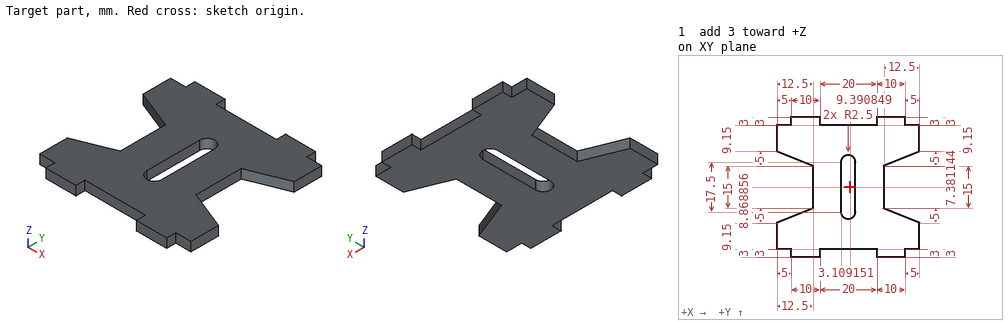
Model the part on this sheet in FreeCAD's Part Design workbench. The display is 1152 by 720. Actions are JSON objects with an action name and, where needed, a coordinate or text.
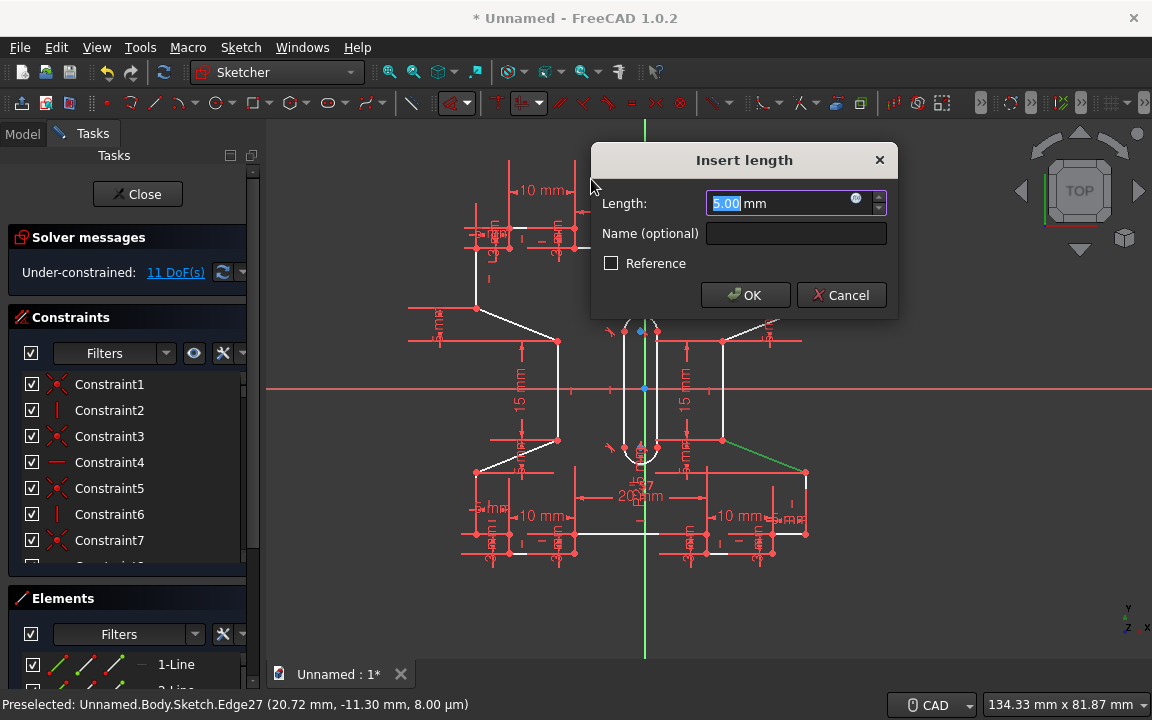
{"action": "type", "text": "5"}
{"action": "key", "text": "Return"}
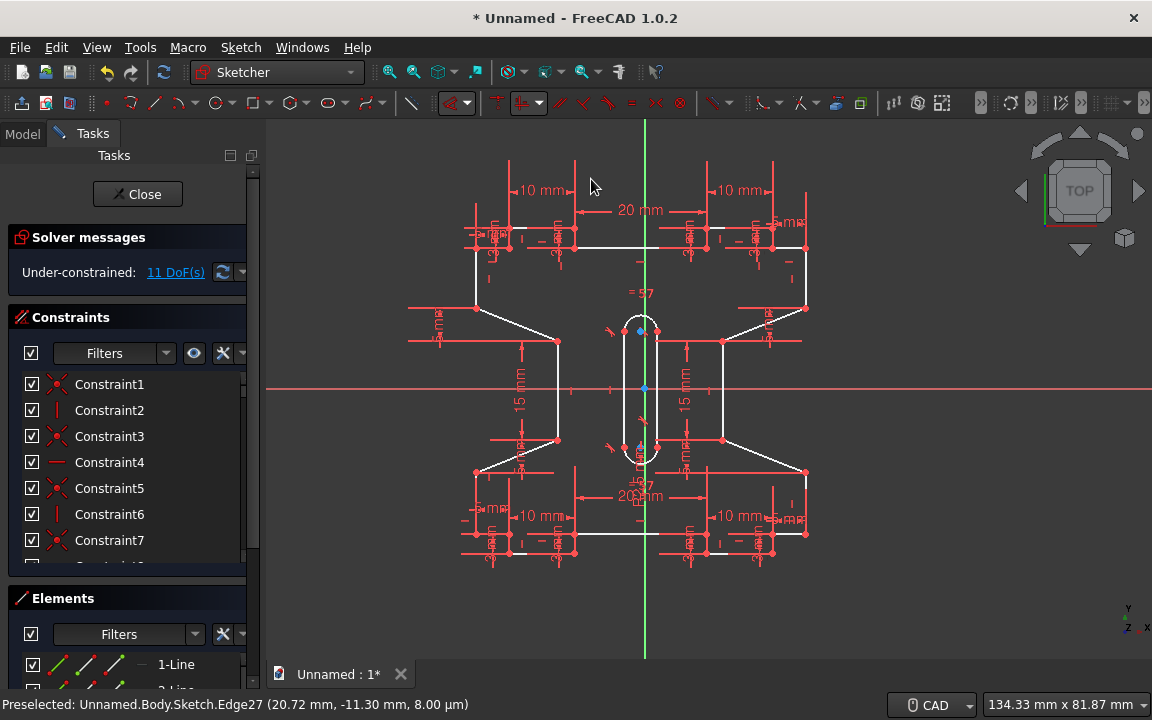
{"action": "left_click", "coordinate": [806, 290]}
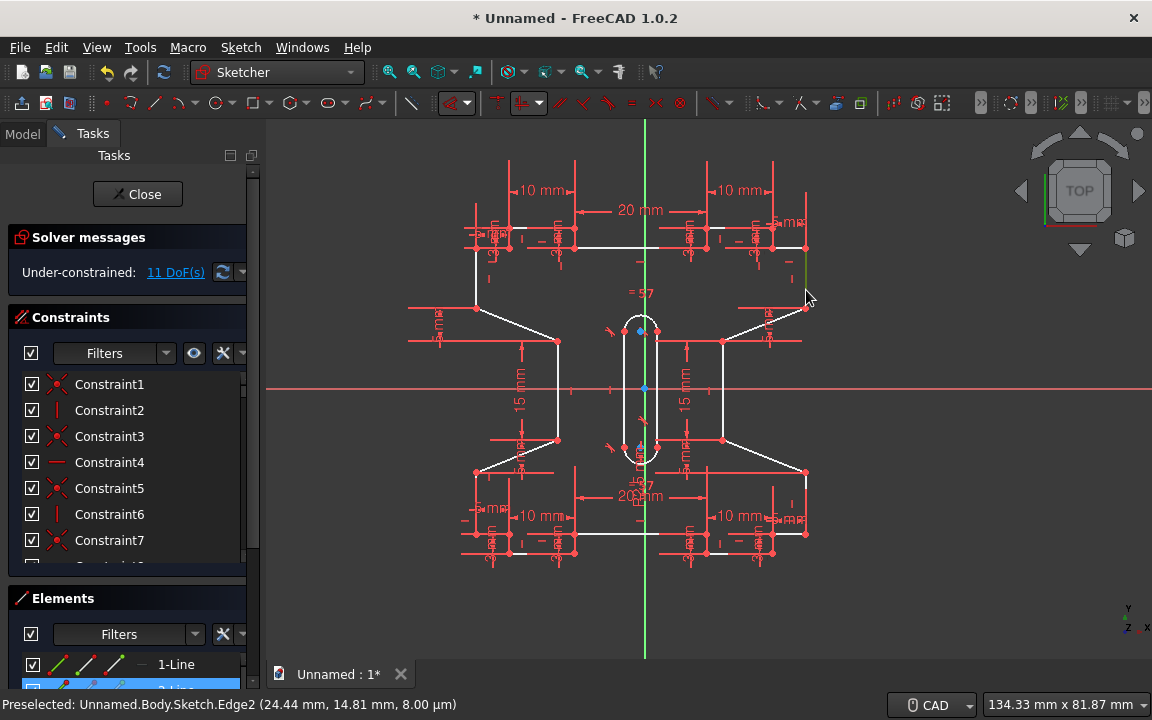
{"action": "left_click", "coordinate": [470, 104]}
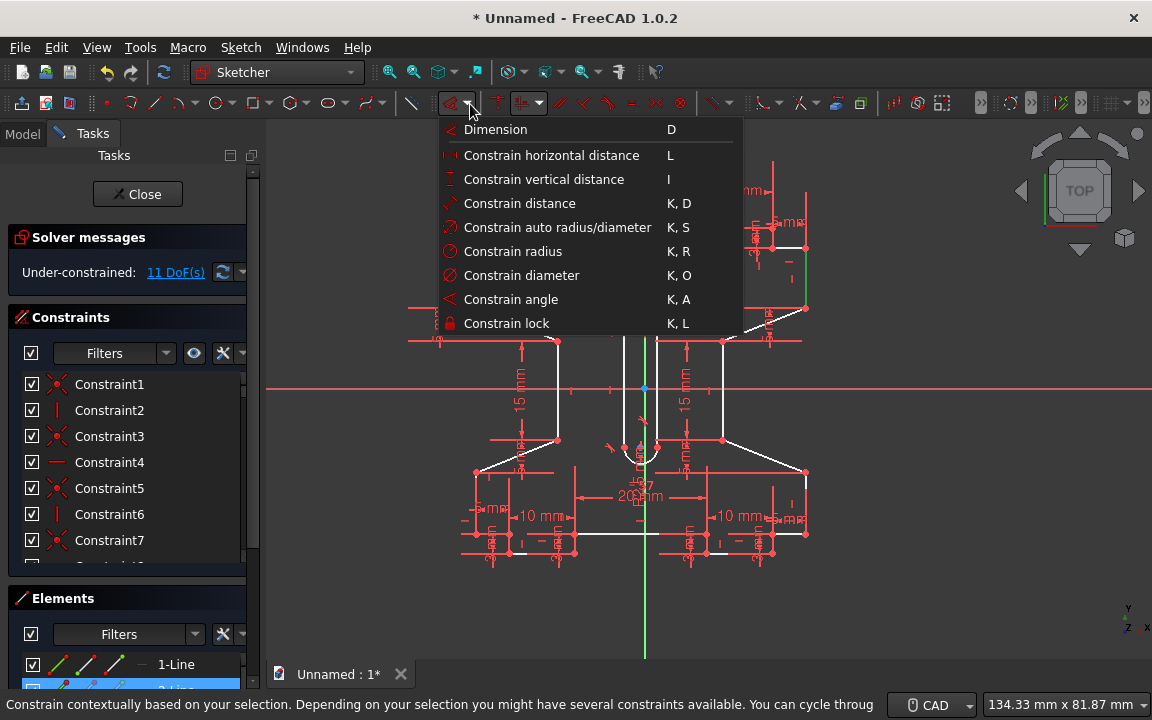
{"action": "left_click", "coordinate": [591, 179]}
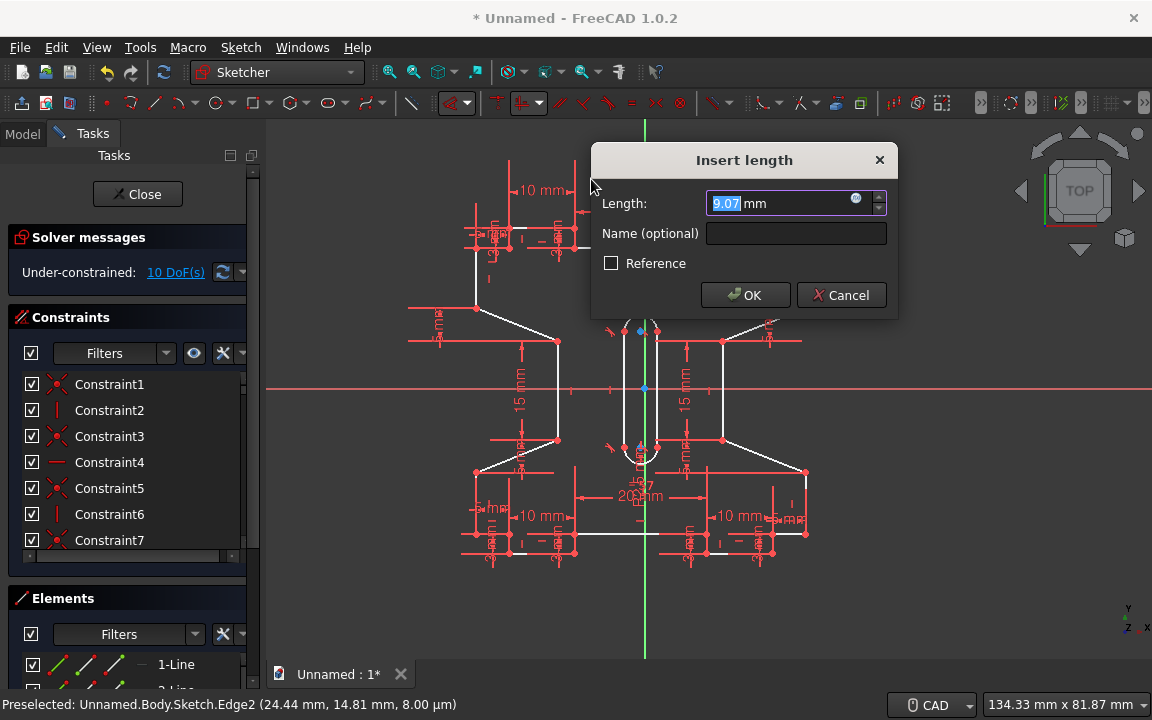
{"action": "type", "text": "9.15"}
{"action": "key", "text": "Return"}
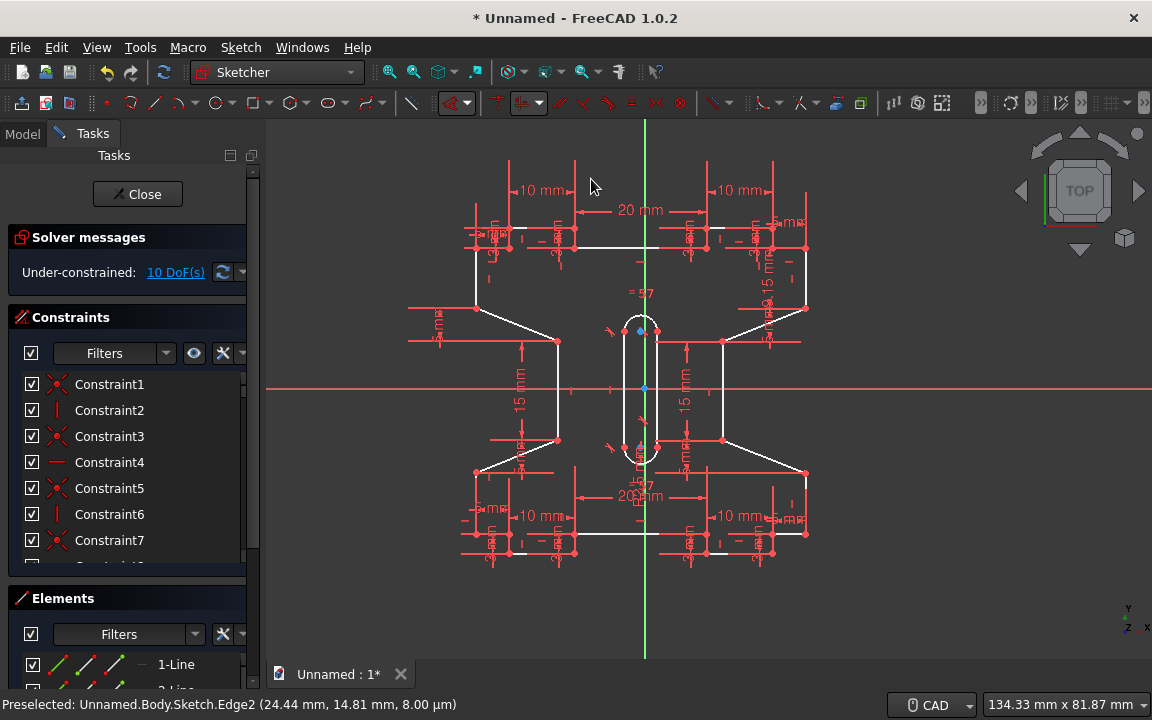
{"action": "left_click", "coordinate": [476, 266]}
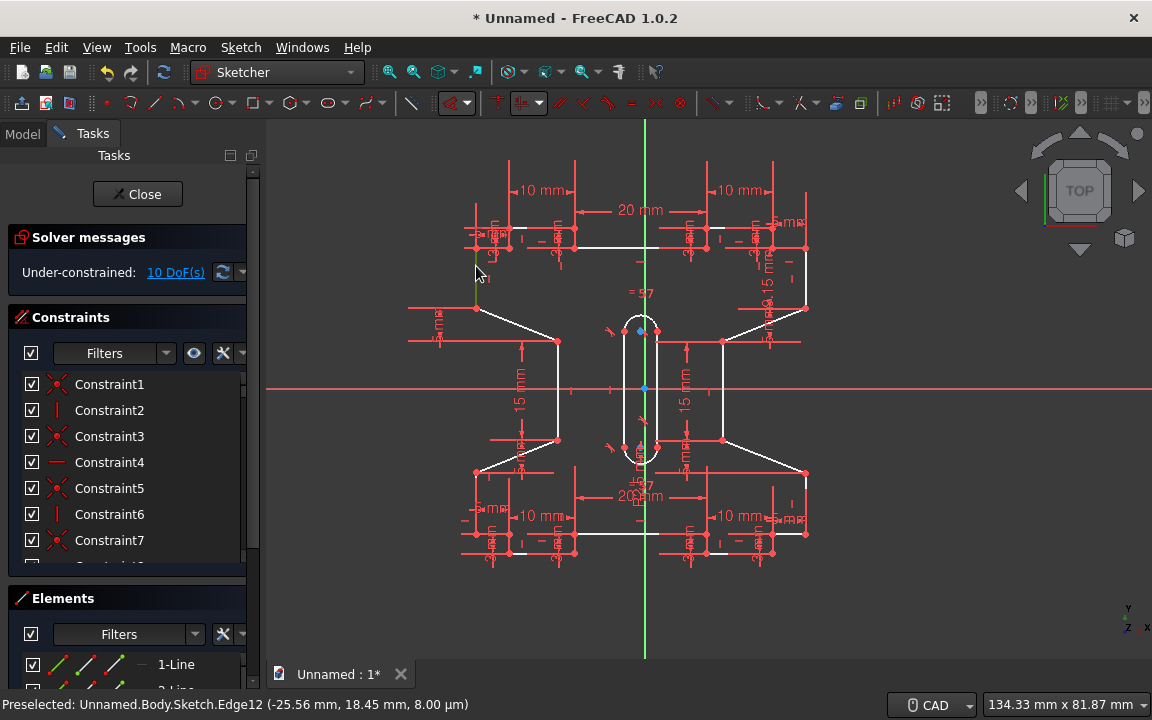
{"action": "key", "text": "i"}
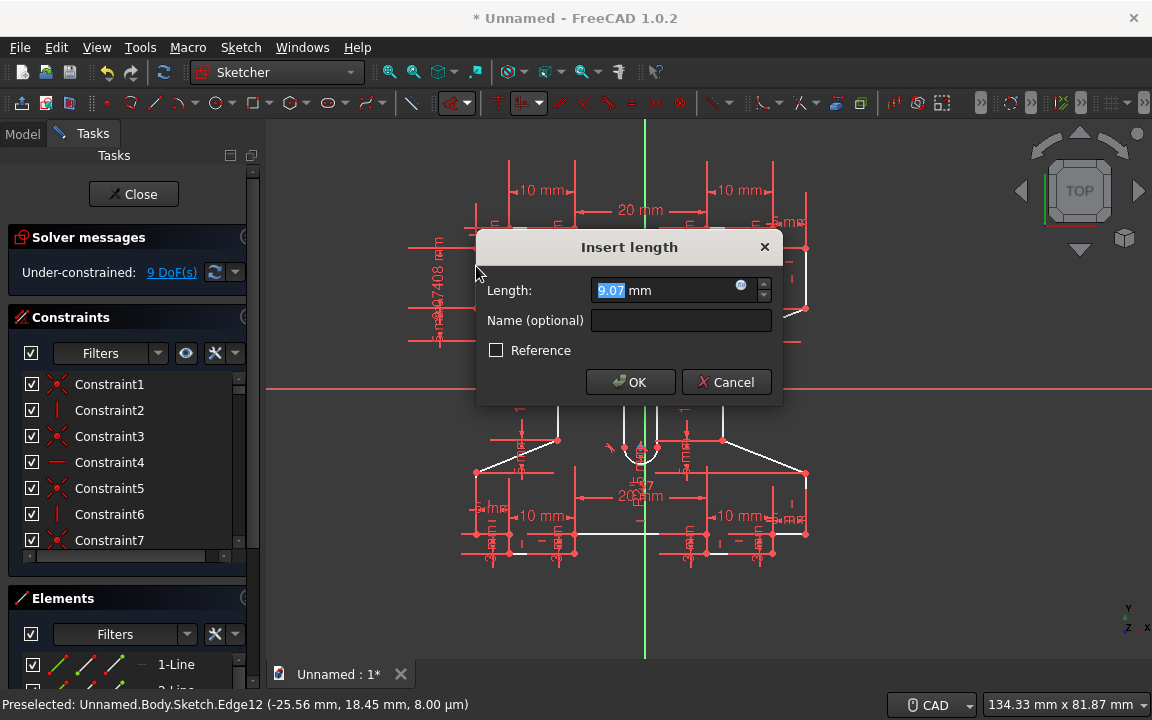
{"action": "type", "text": "9.15"}
{"action": "key", "text": "Return"}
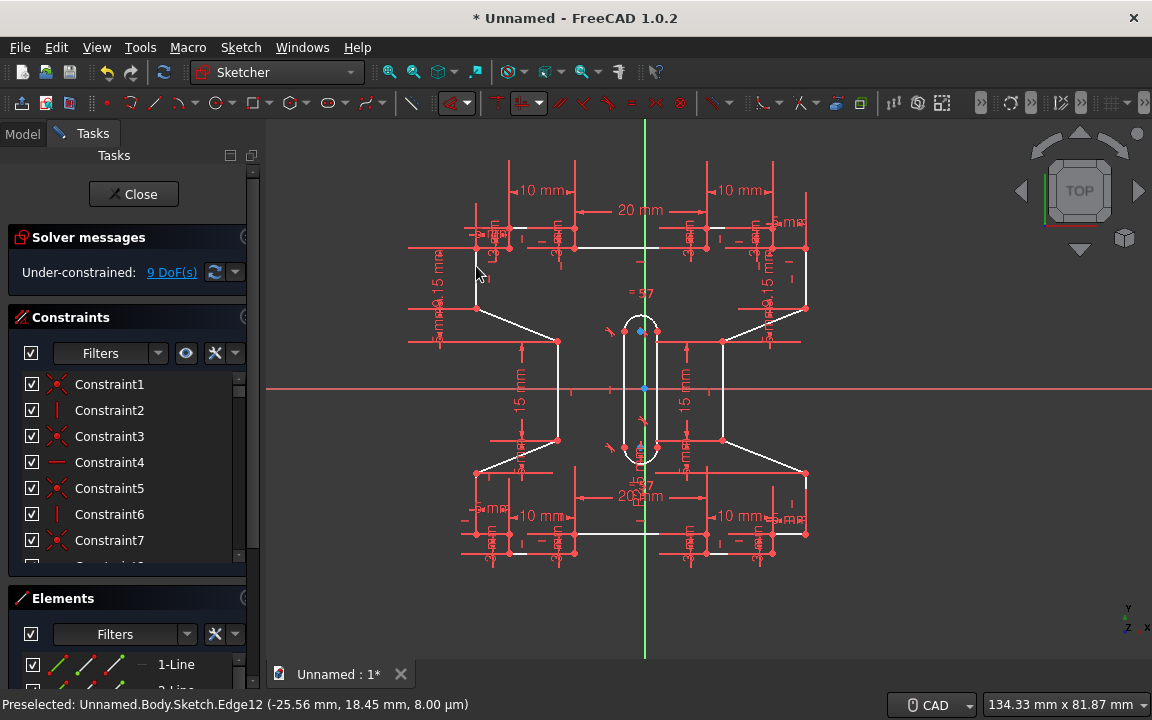
{"action": "left_click", "coordinate": [476, 492]}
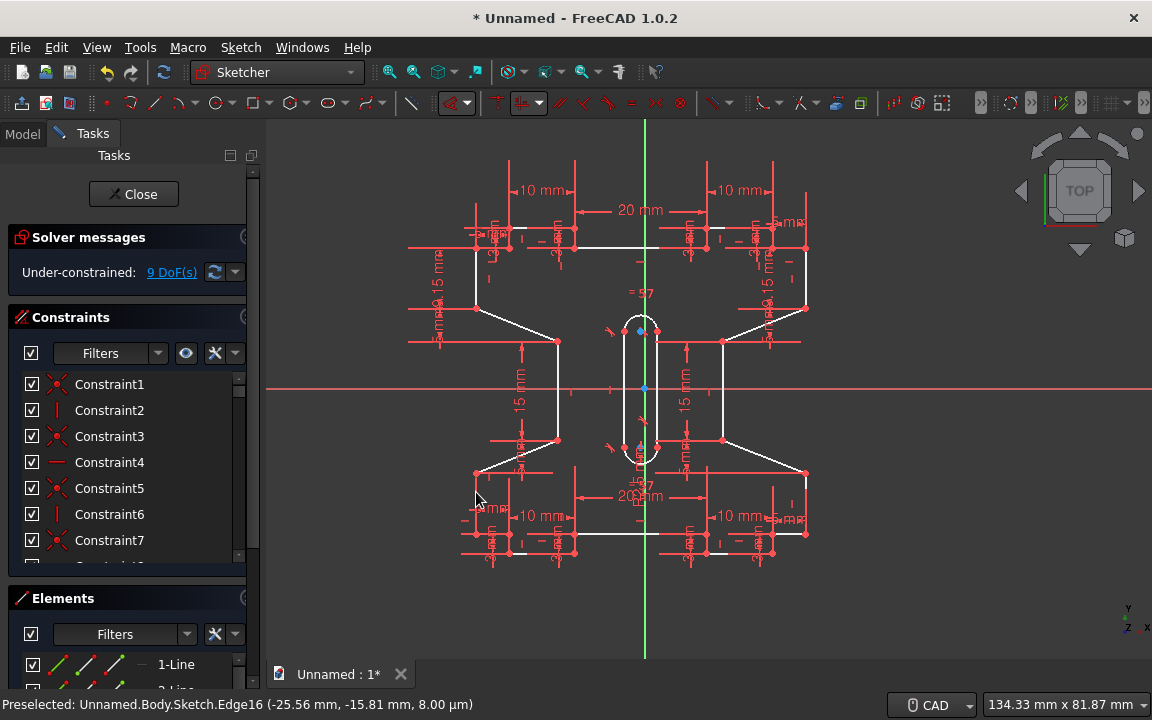
{"action": "key", "text": "i"}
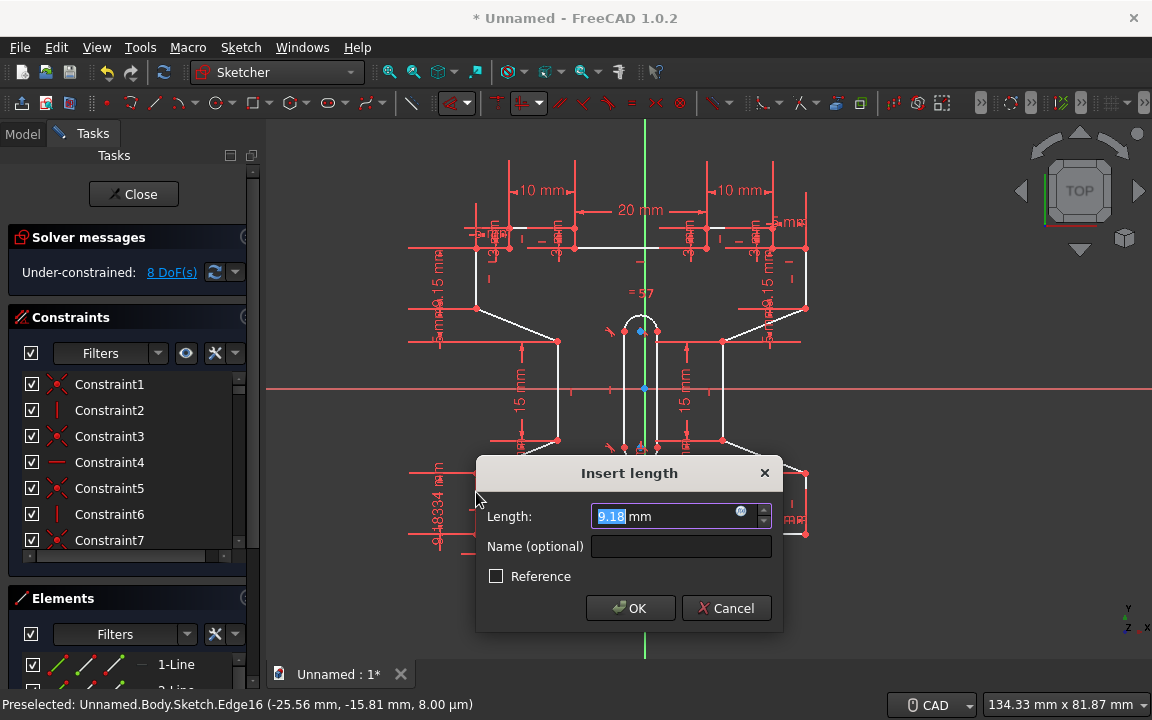
{"action": "type", "text": "9.15"}
{"action": "key", "text": "Return"}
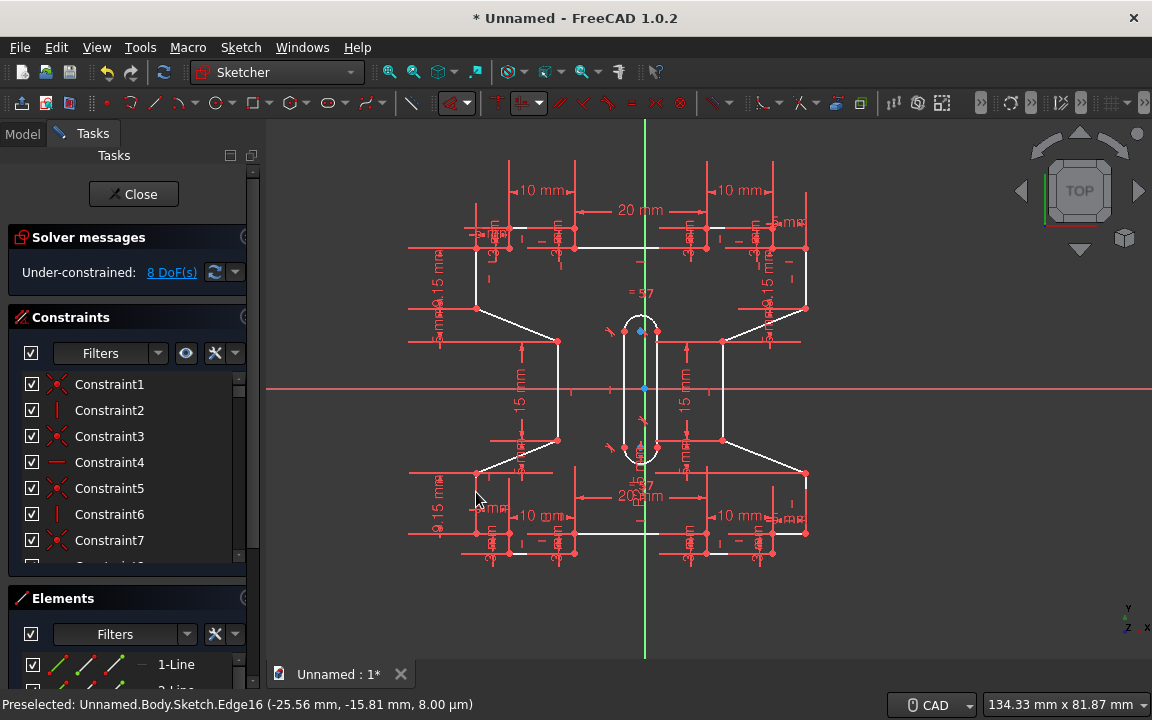
{"action": "left_click", "coordinate": [624, 413]}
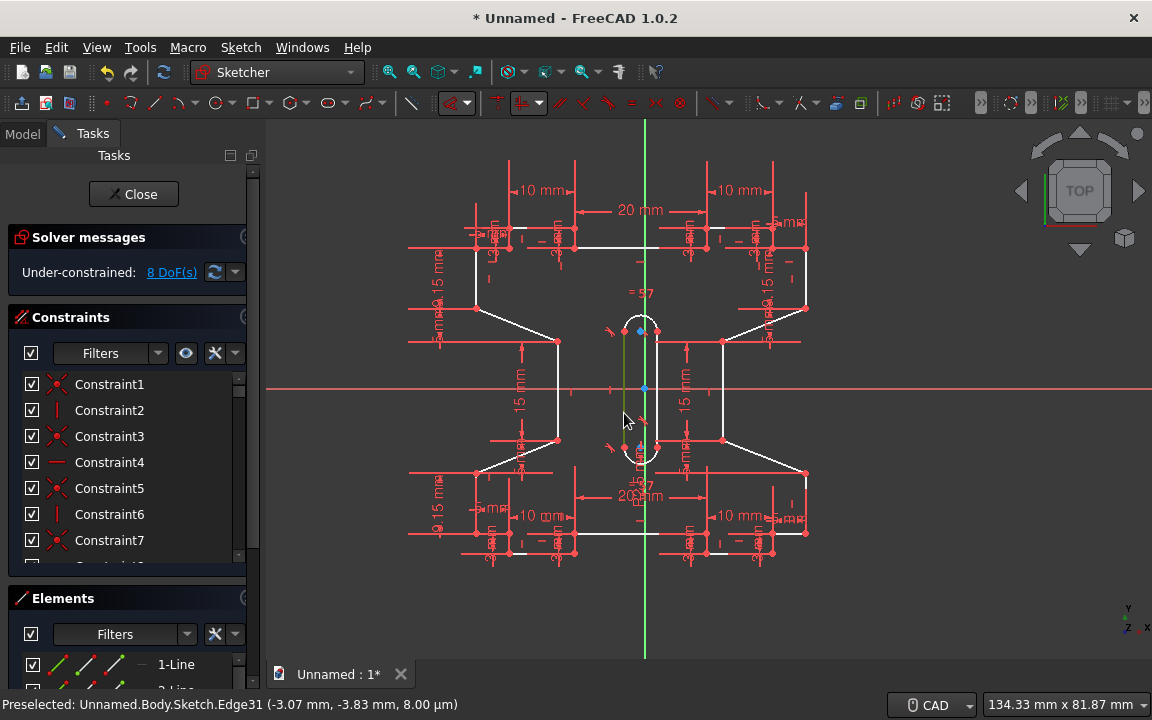
{"action": "left_click", "coordinate": [470, 104]}